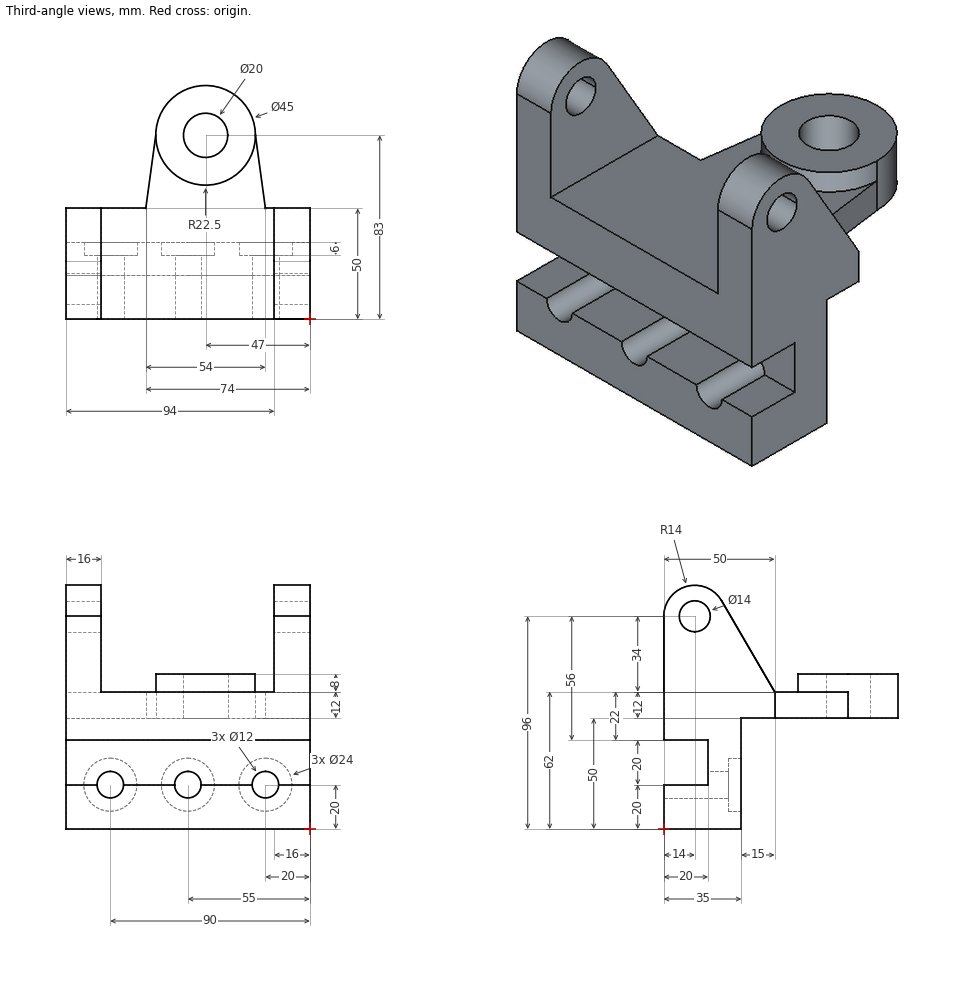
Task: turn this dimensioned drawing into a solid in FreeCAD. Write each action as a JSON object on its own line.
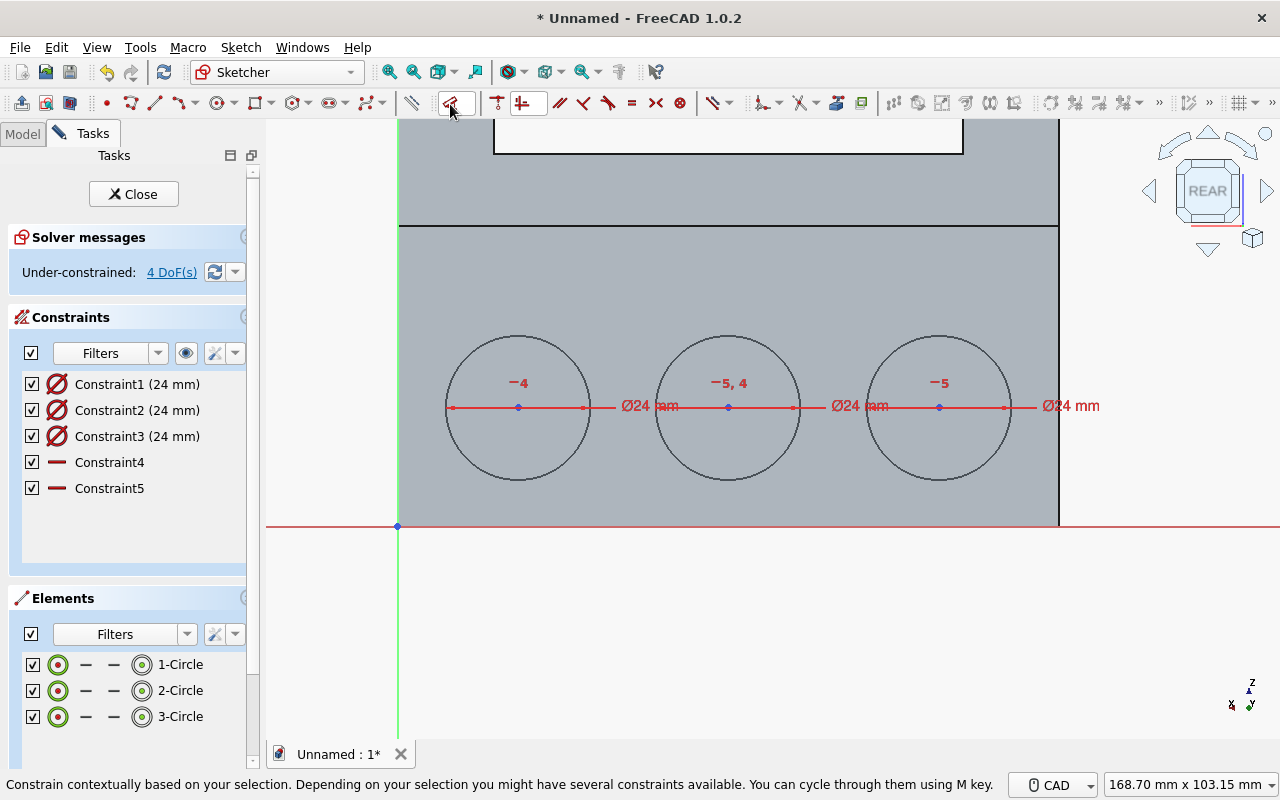
{"action": "left_click", "coordinate": [518, 408]}
{"action": "left_click", "coordinate": [458, 561]}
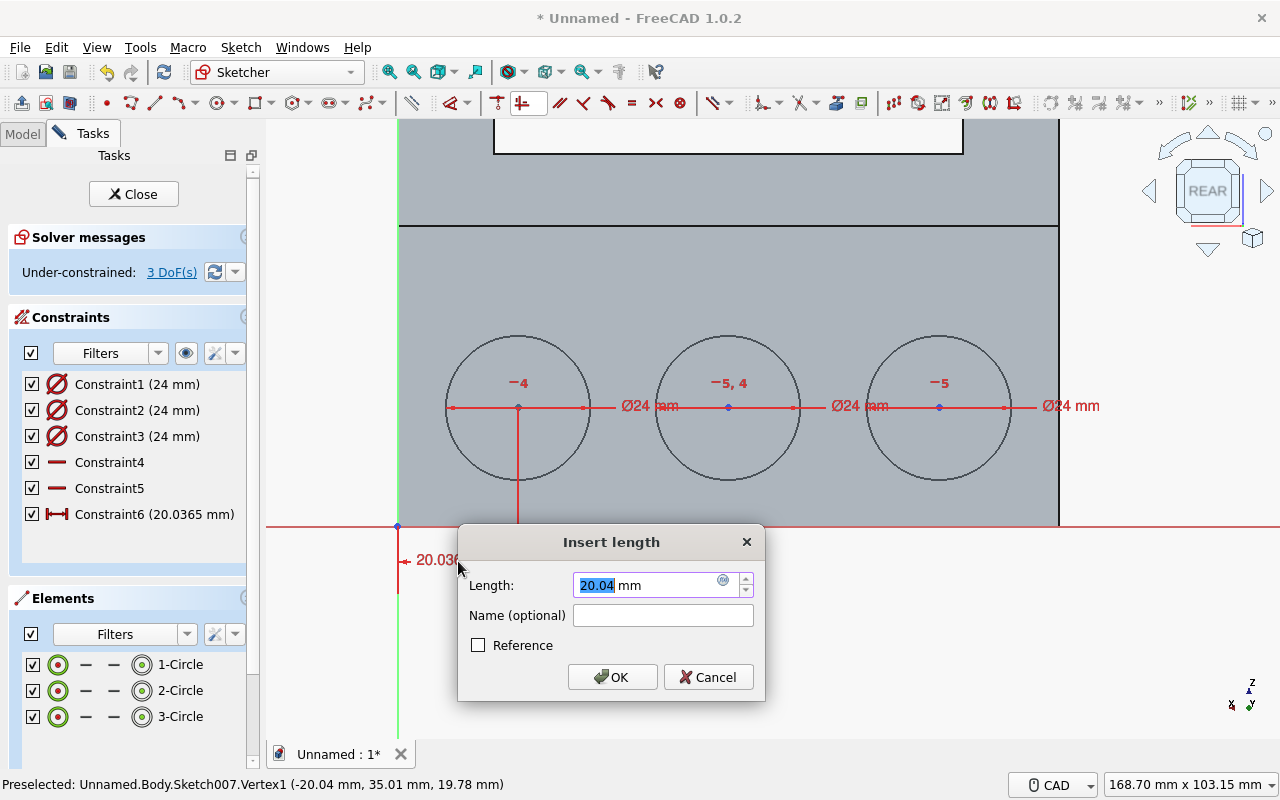
{"action": "type", "text": "20"}
{"action": "key", "text": "Return"}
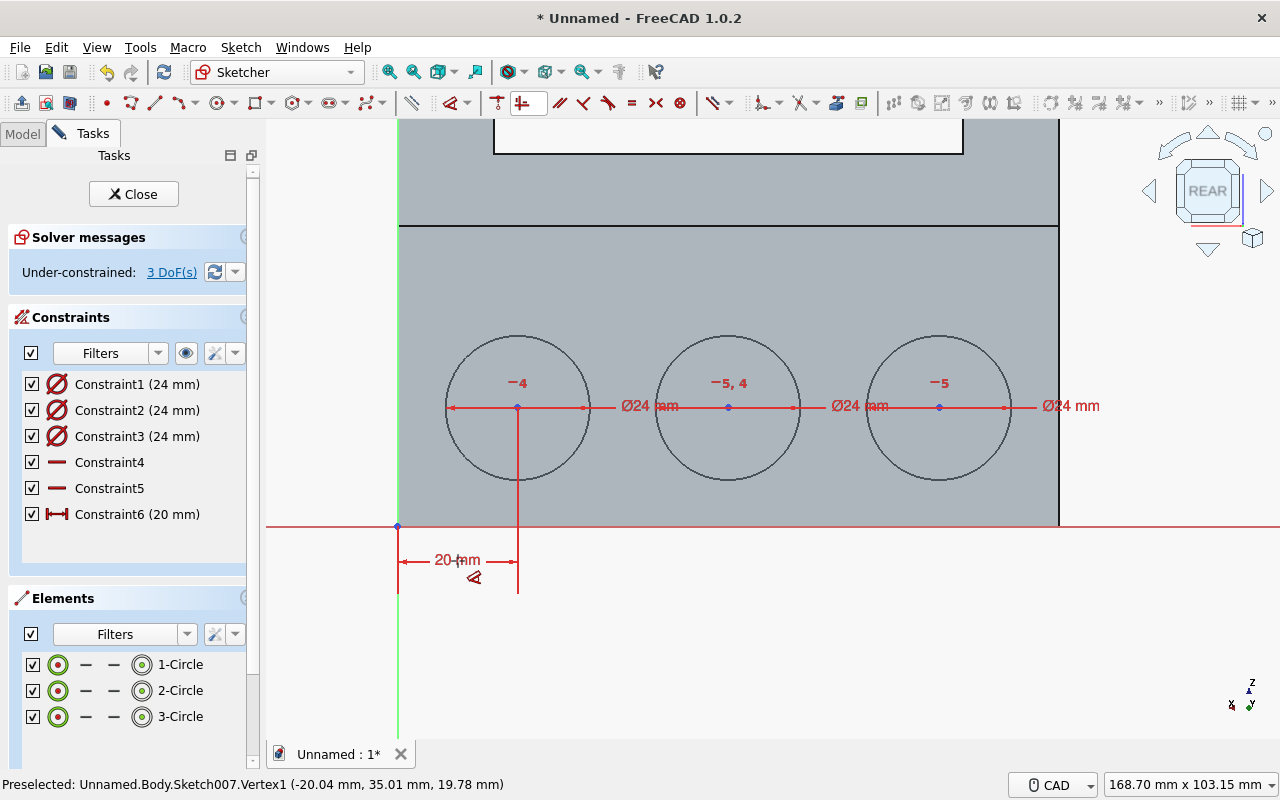
{"action": "left_click", "coordinate": [518, 408]}
{"action": "left_click", "coordinate": [364, 467]}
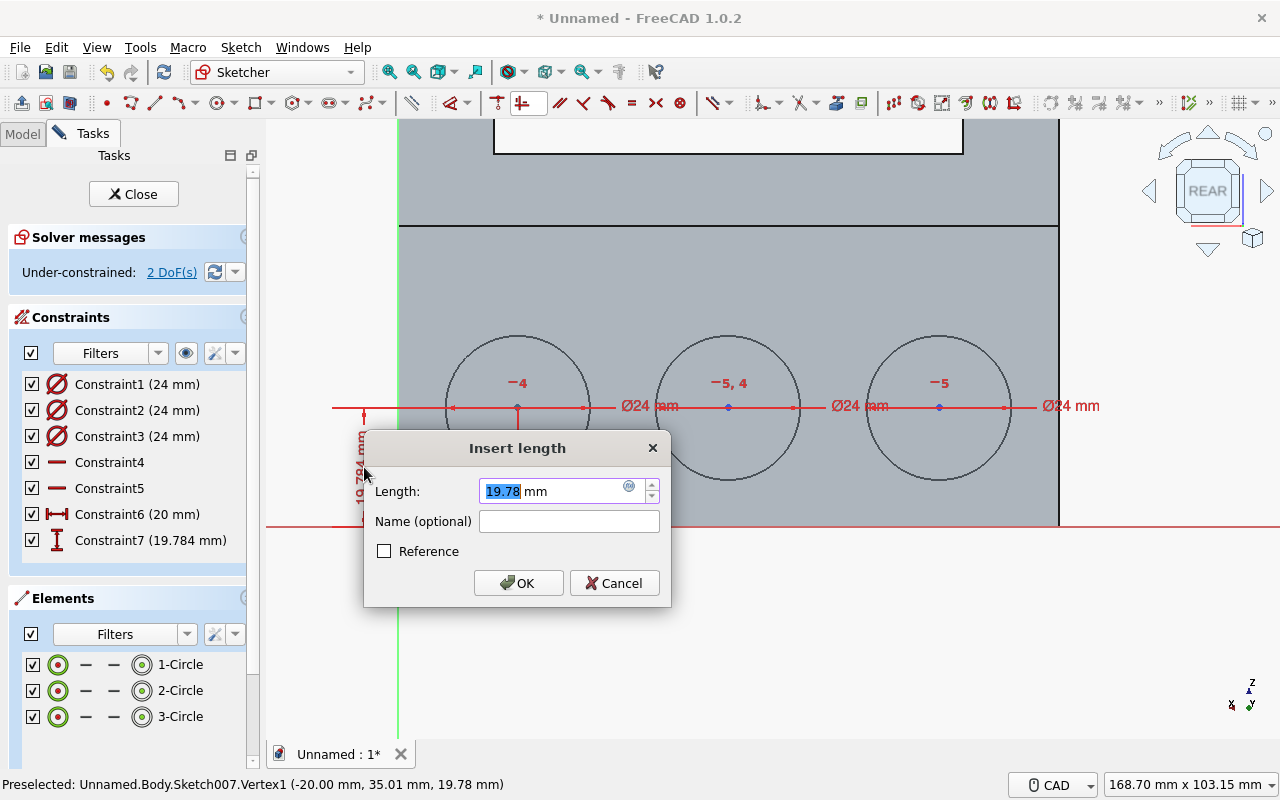
{"action": "type", "text": "20"}
{"action": "key", "text": "Return"}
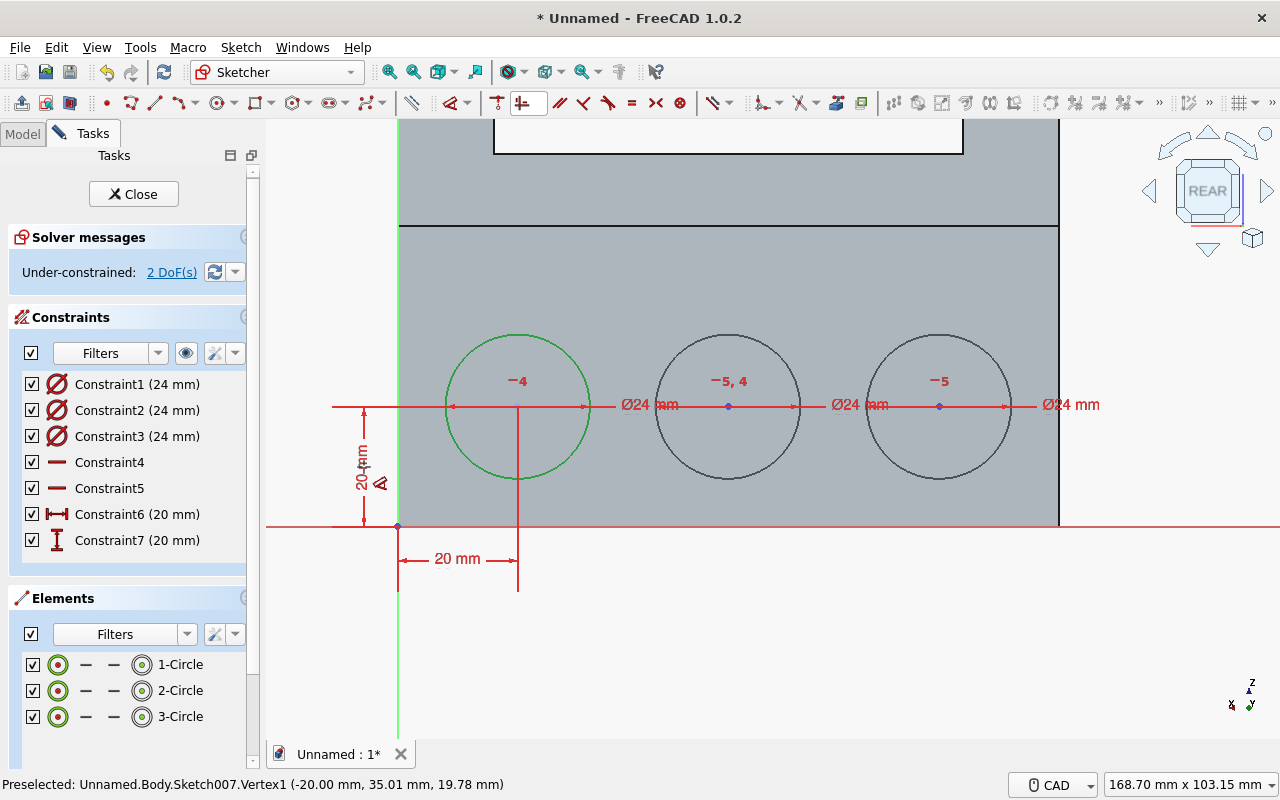
{"action": "left_click", "coordinate": [728, 407]}
{"action": "left_click", "coordinate": [563, 561]}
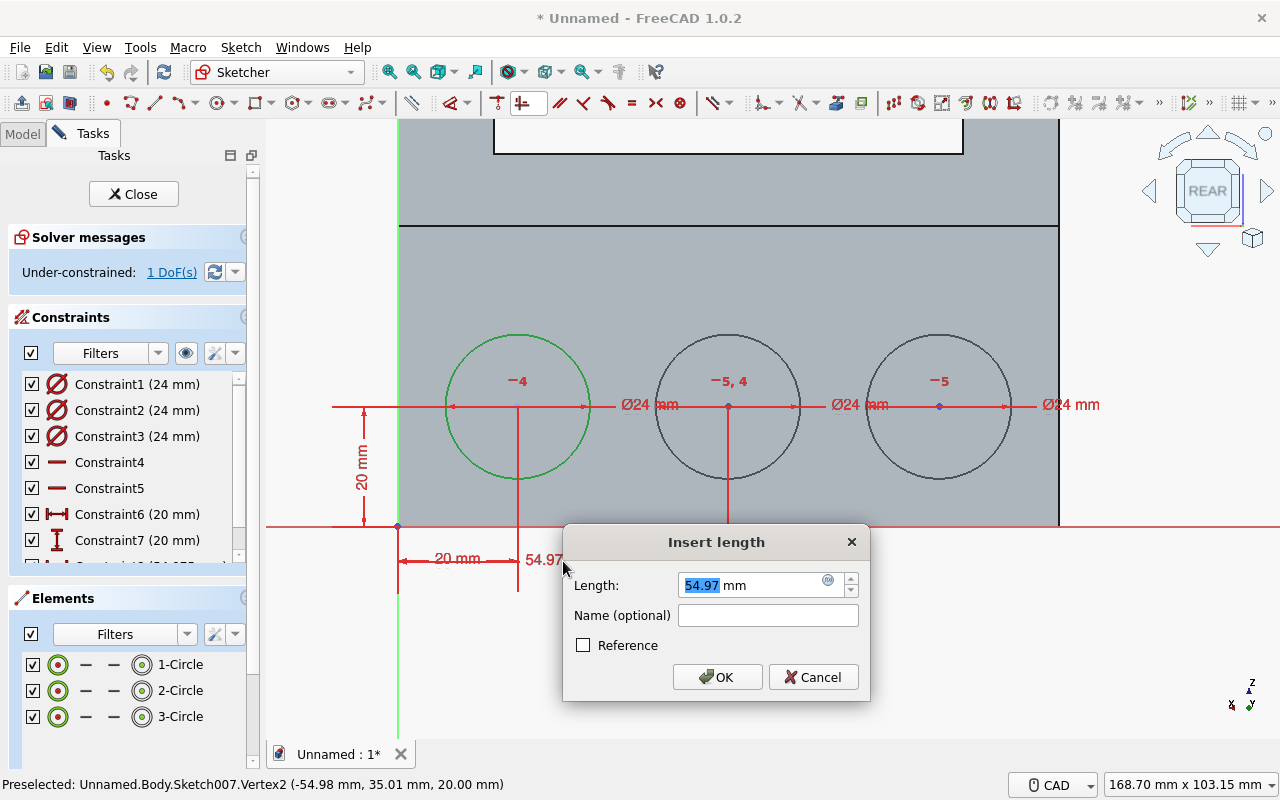
{"action": "type", "text": "55"}
{"action": "key", "text": "Return"}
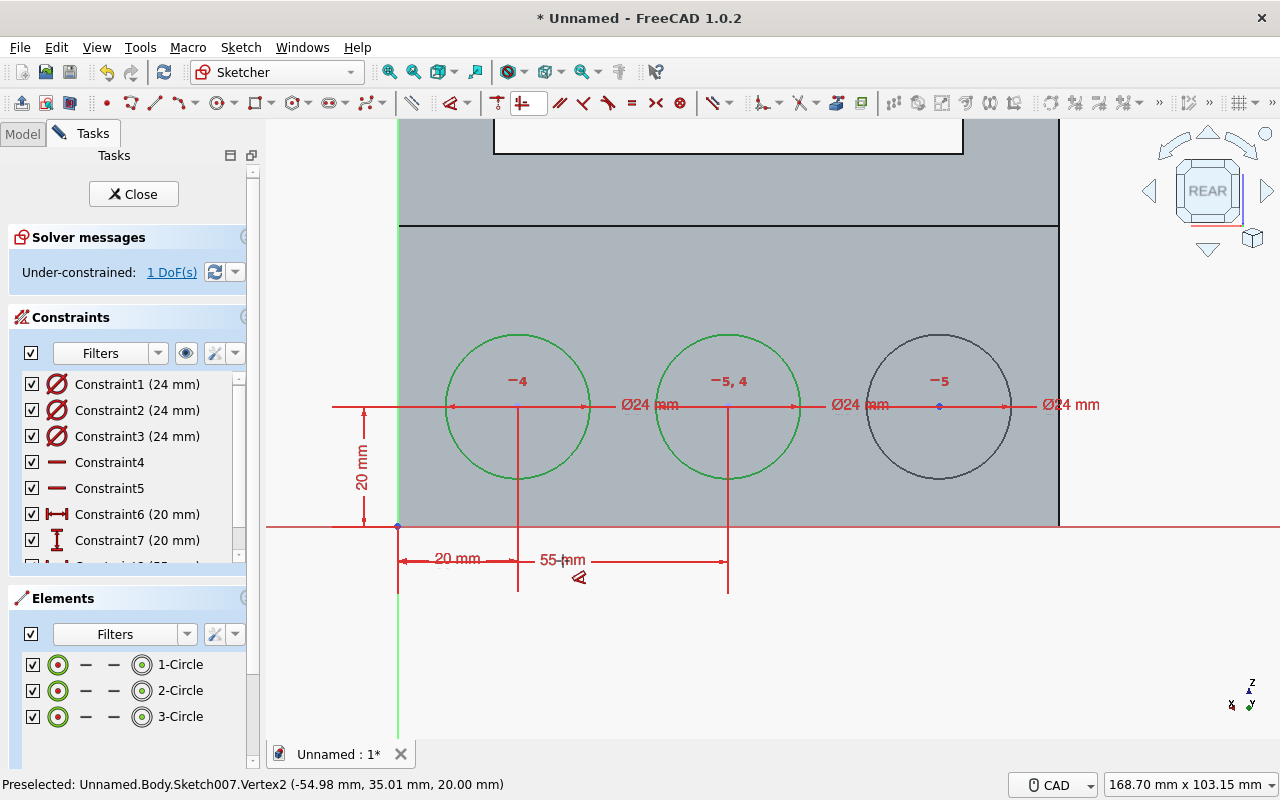
{"action": "left_click", "coordinate": [939, 407]}
{"action": "left_click", "coordinate": [668, 561]}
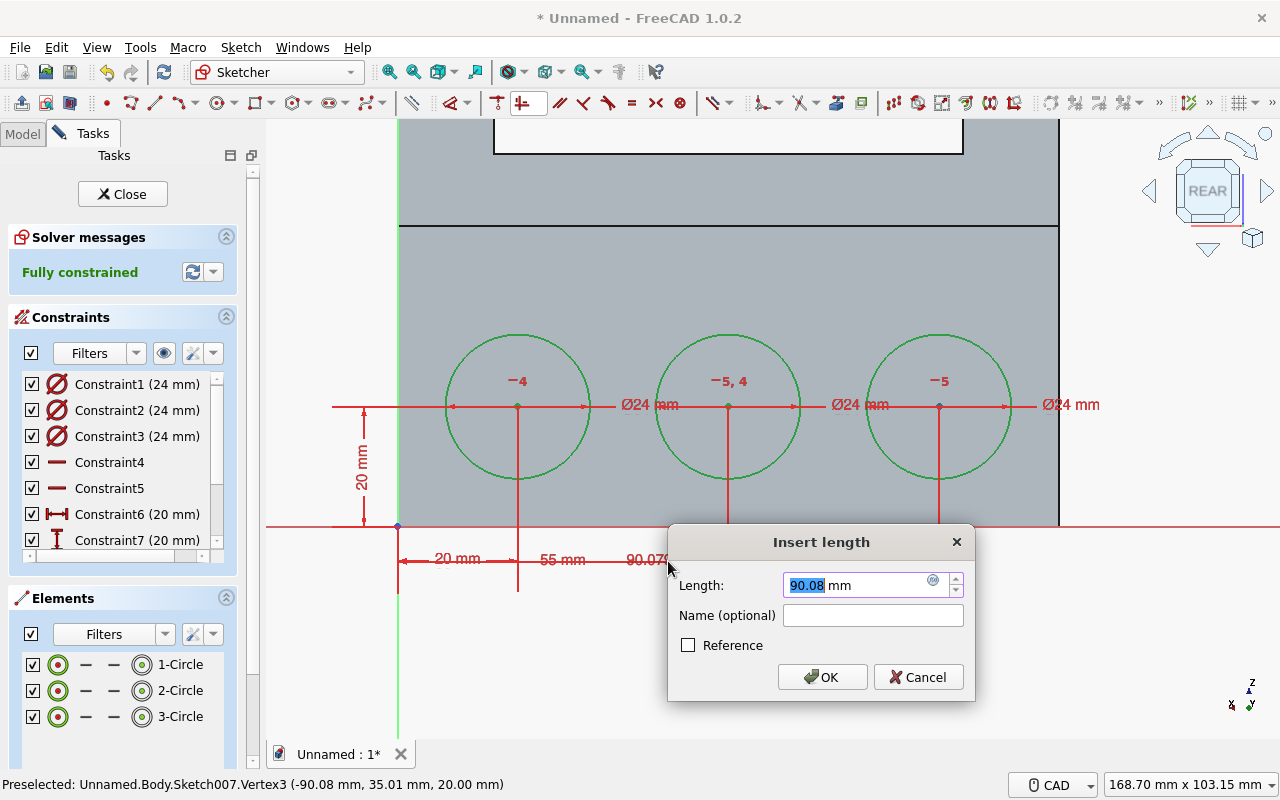
{"action": "type", "text": "90"}
{"action": "key", "text": "Return"}
{"action": "key", "text": "Escape"}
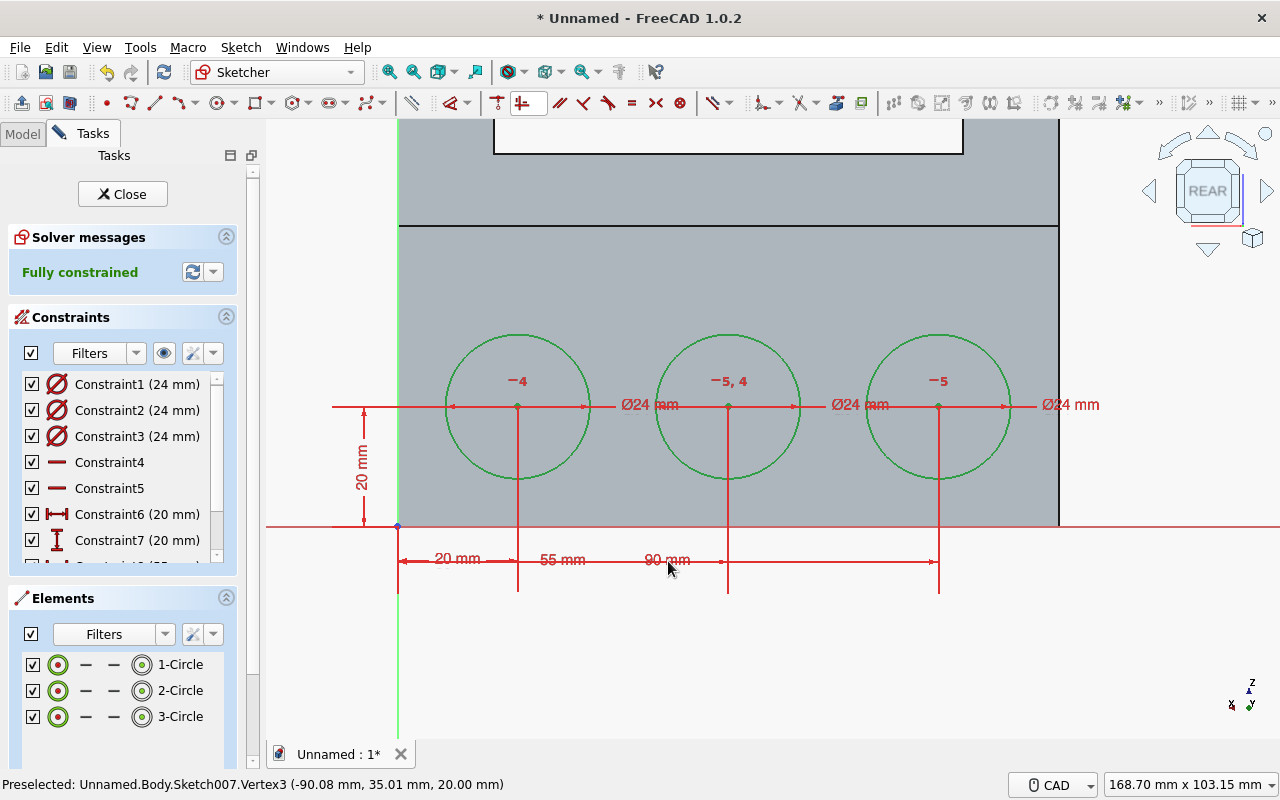
{"action": "left_click", "coordinate": [123, 194]}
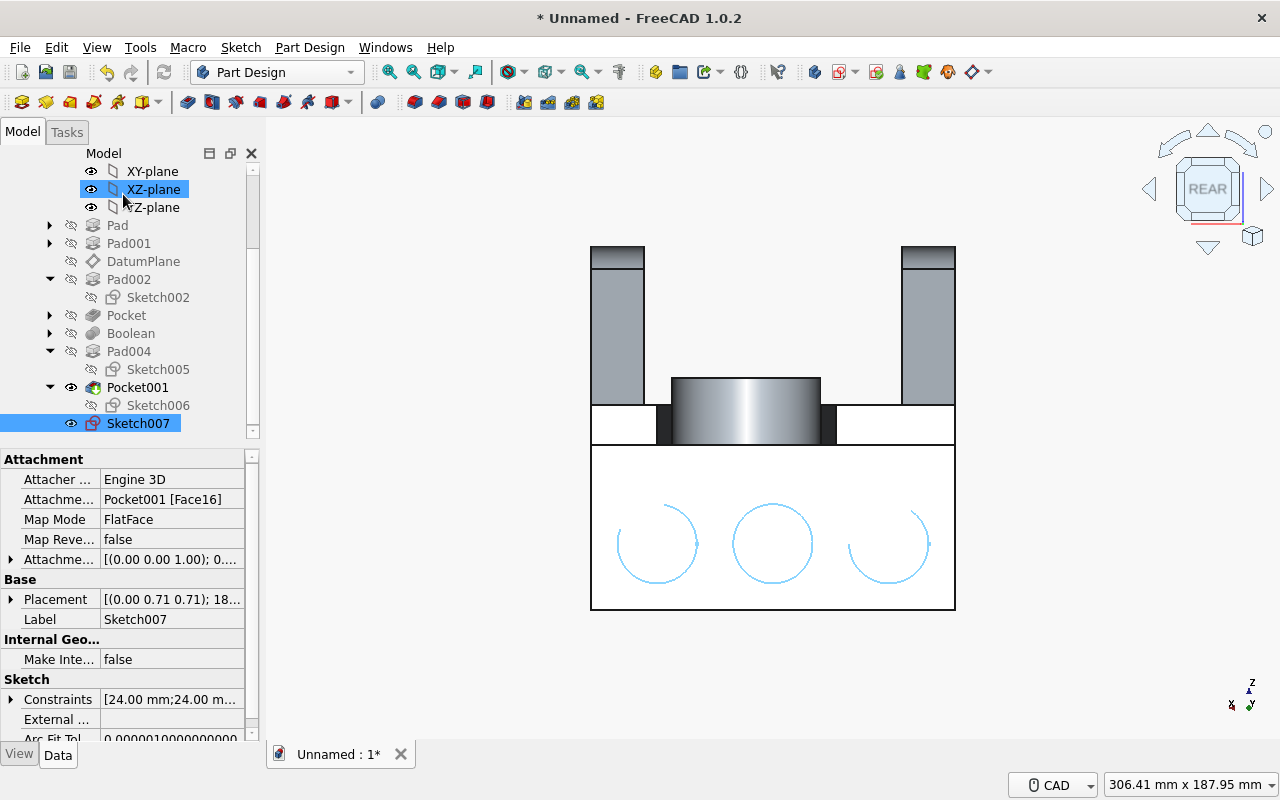
{"action": "left_click", "coordinate": [188, 102]}